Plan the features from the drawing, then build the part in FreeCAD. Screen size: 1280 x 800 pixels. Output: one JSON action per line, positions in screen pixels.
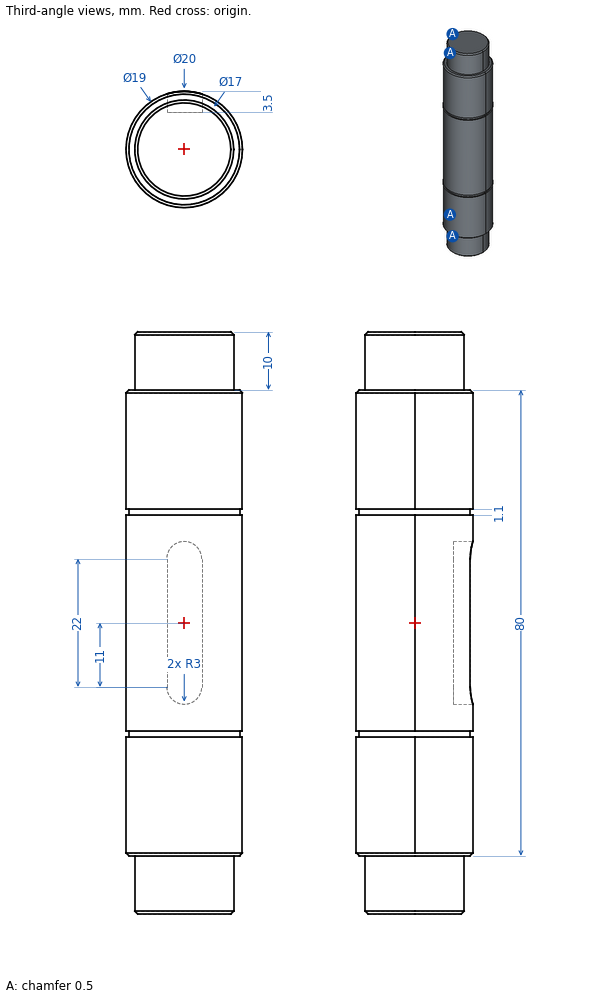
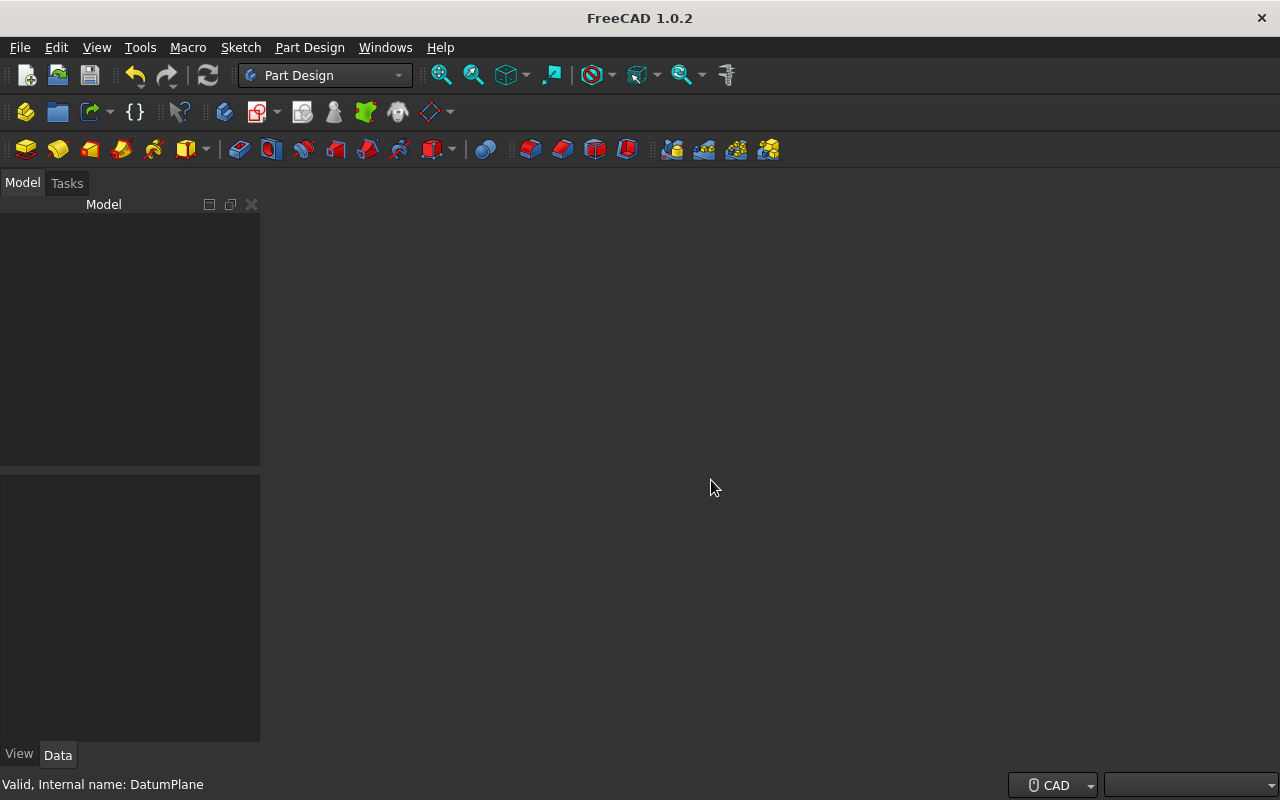
{"action": "left_click", "coordinate": [26, 76]}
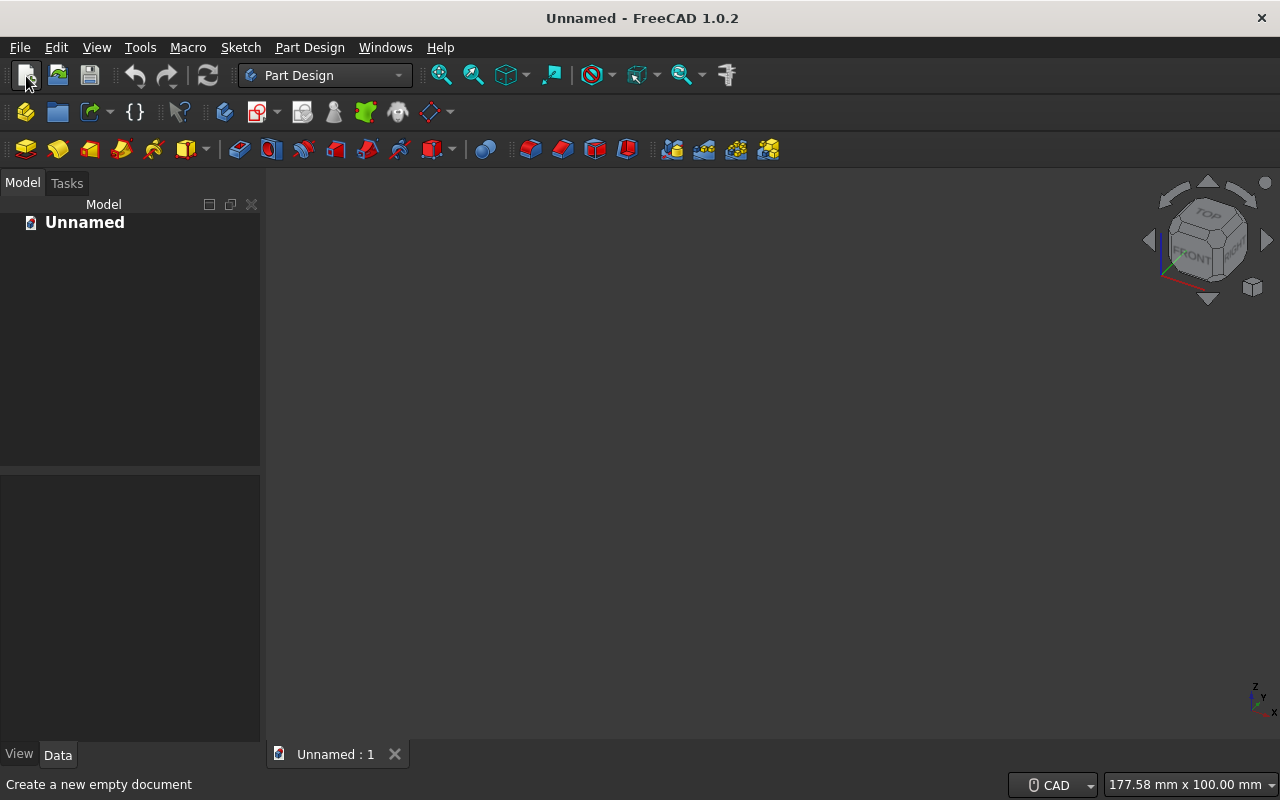
{"action": "left_click", "coordinate": [258, 112]}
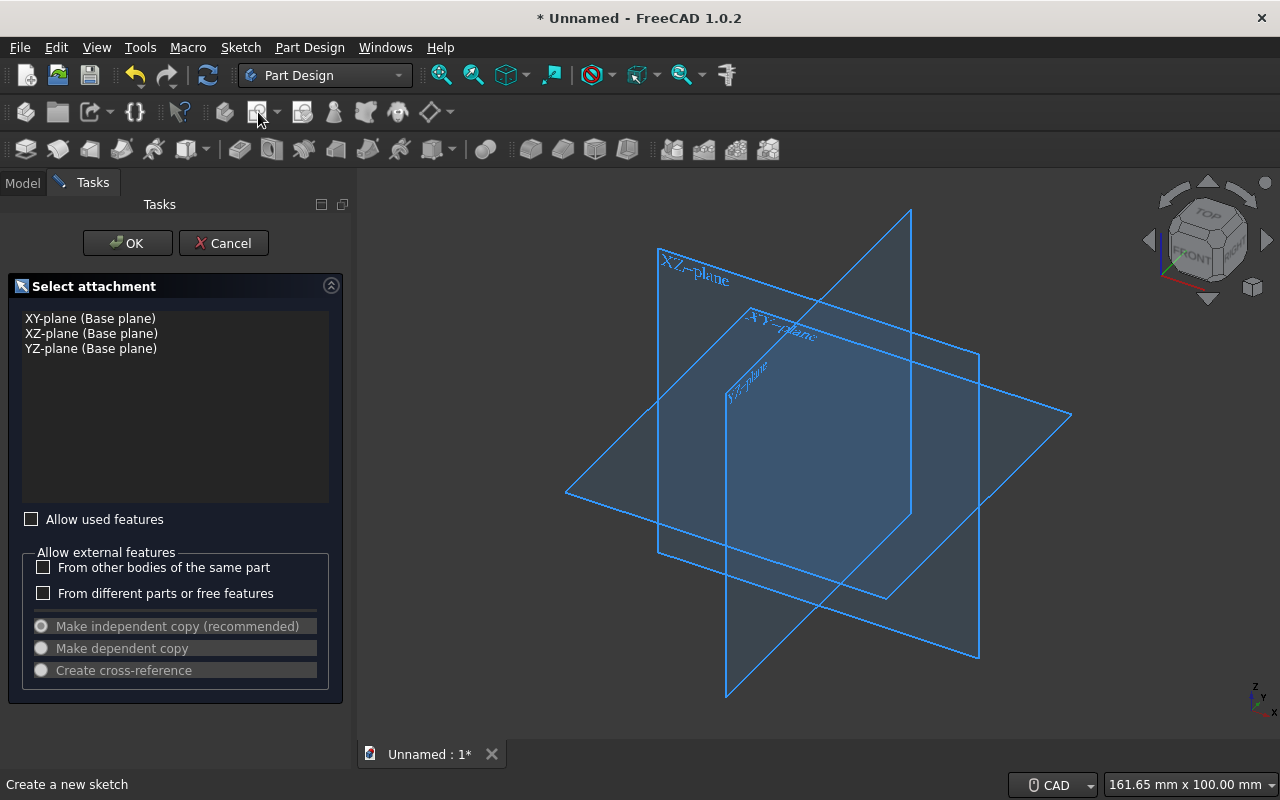
{"action": "left_click", "coordinate": [82, 318]}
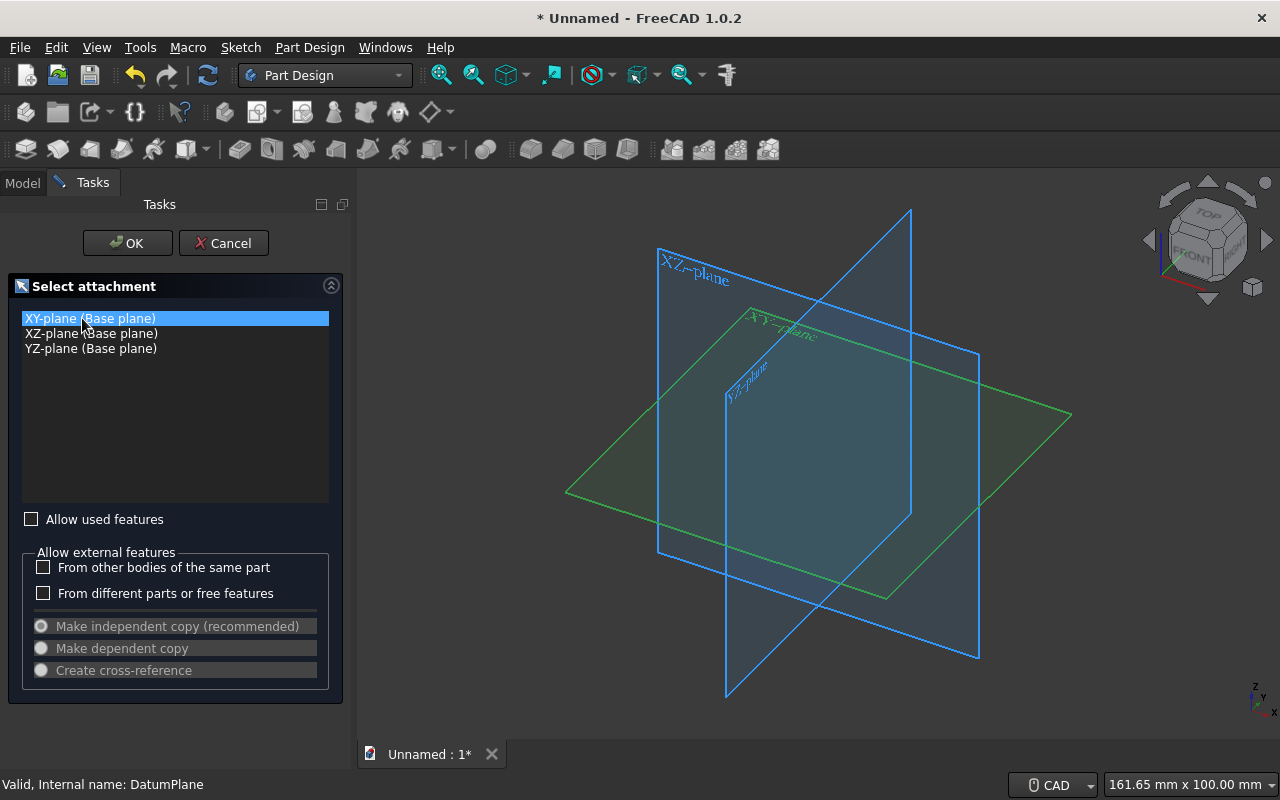
{"action": "left_click", "coordinate": [128, 243]}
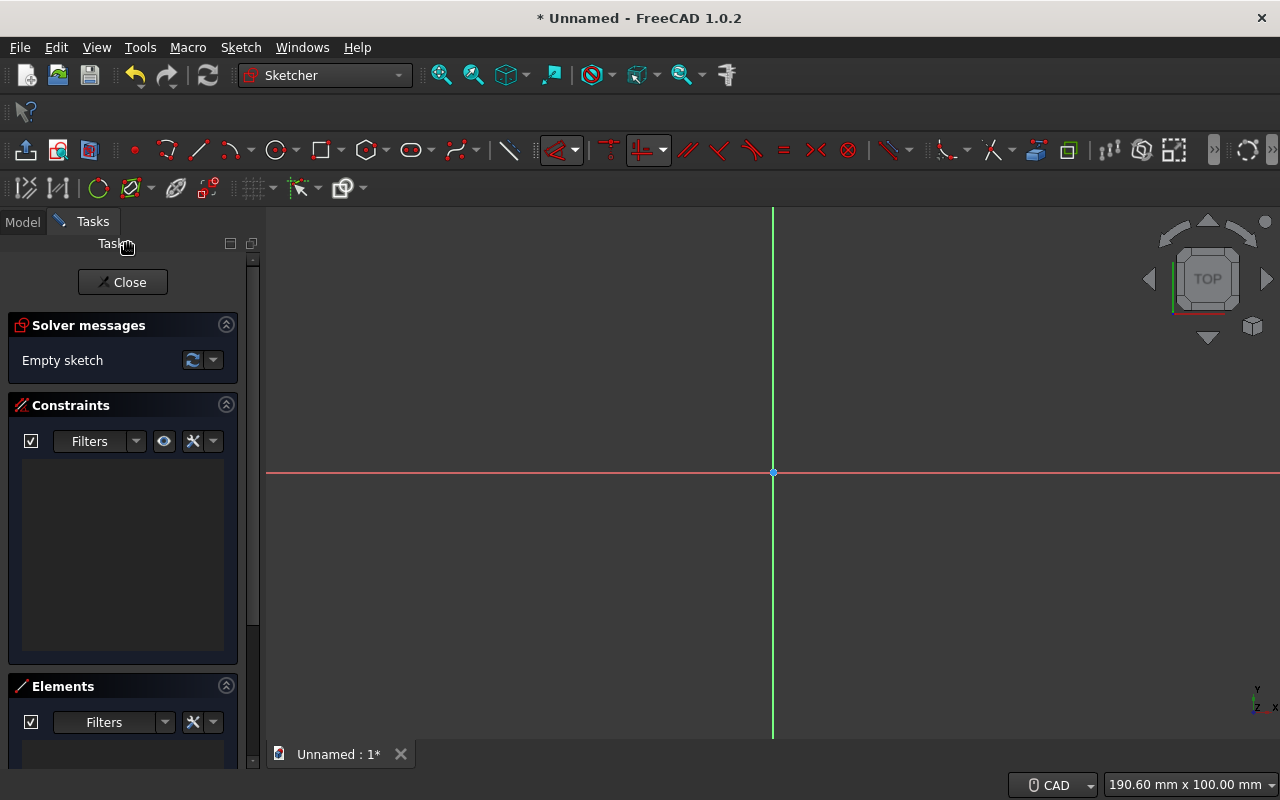
{"action": "scroll", "coordinate": [803, 473], "scroll_direction": "up", "scroll_amount": 6}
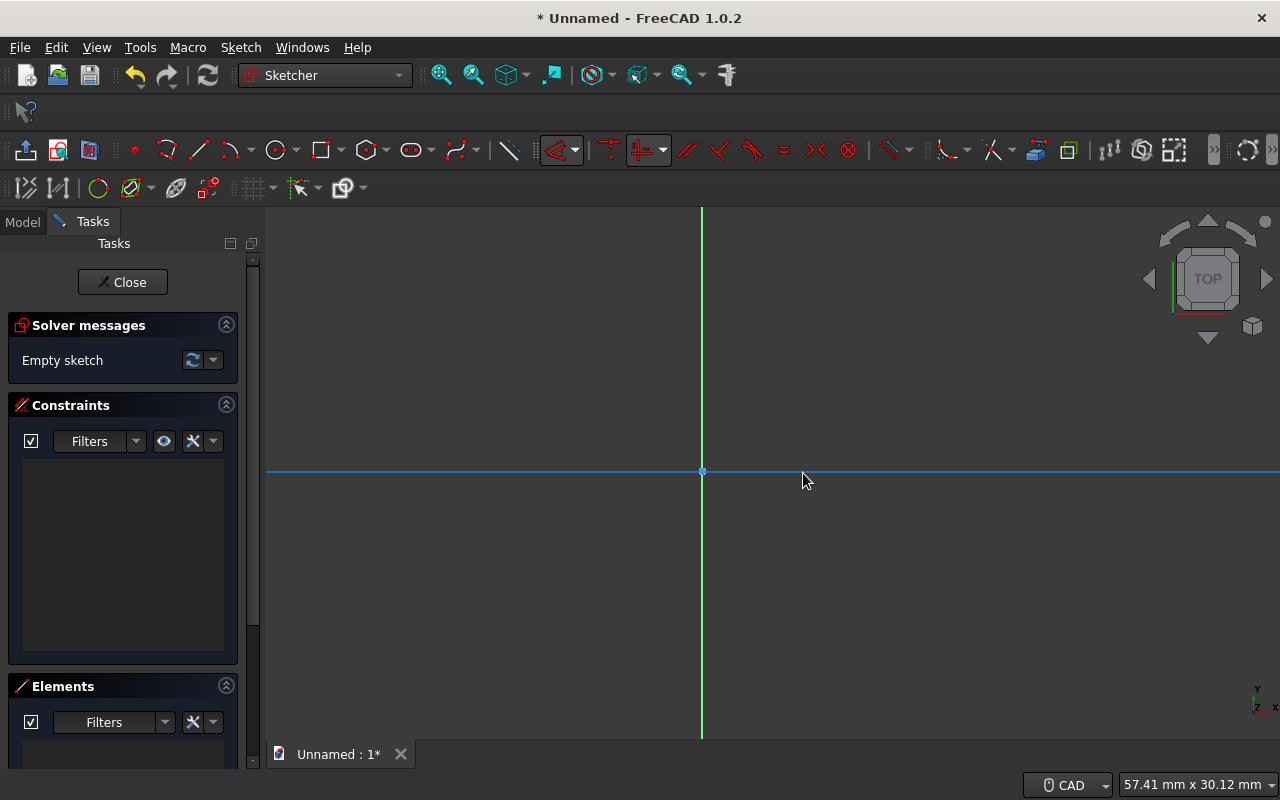
{"action": "key", "text": "g c"}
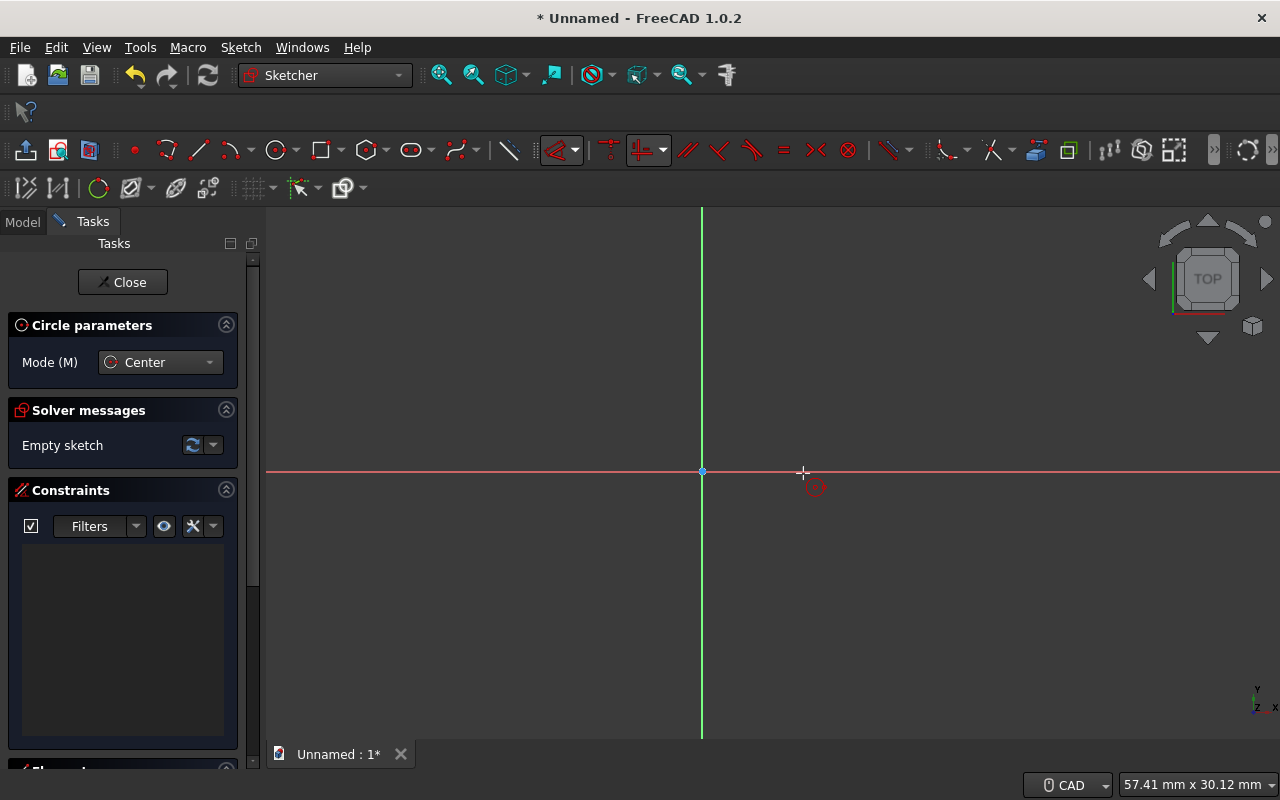
{"action": "left_click", "coordinate": [702, 472]}
{"action": "left_click", "coordinate": [827, 347]}
{"action": "key", "text": "Escape"}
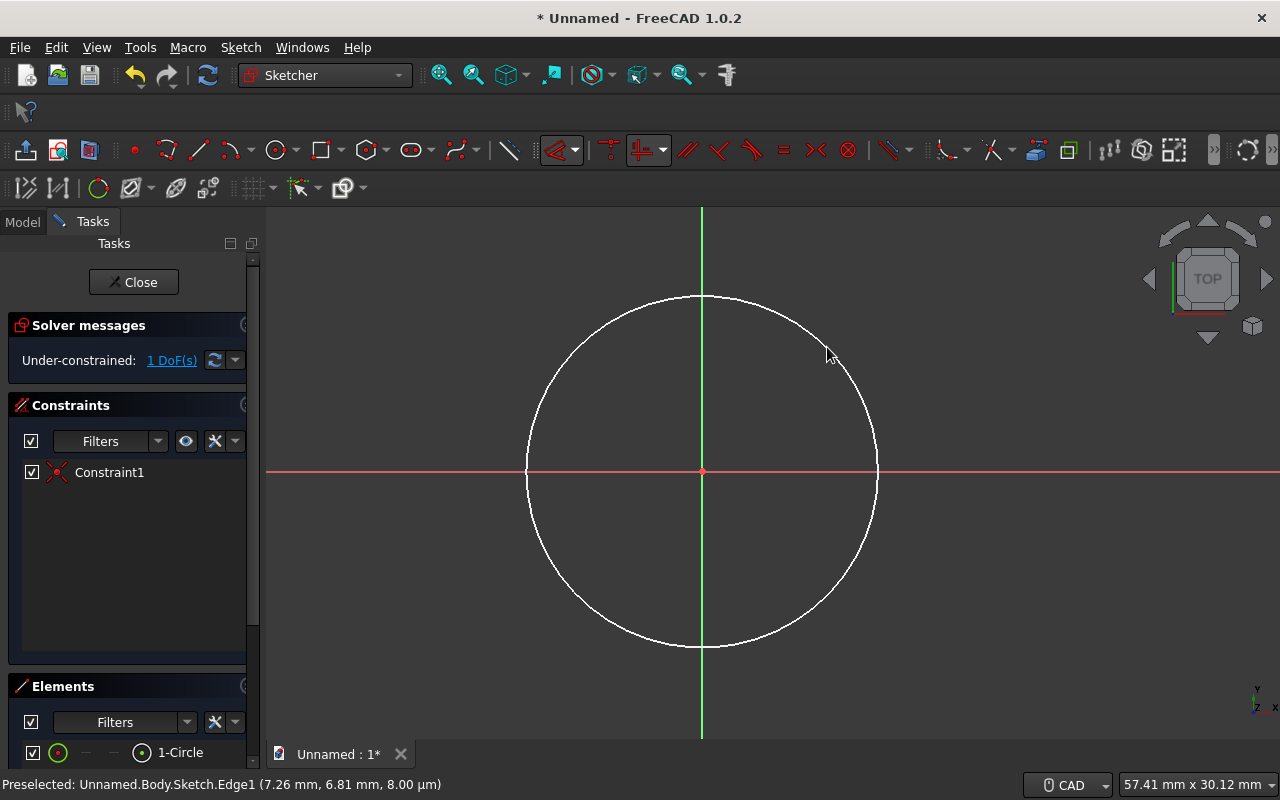
{"action": "key", "text": "d"}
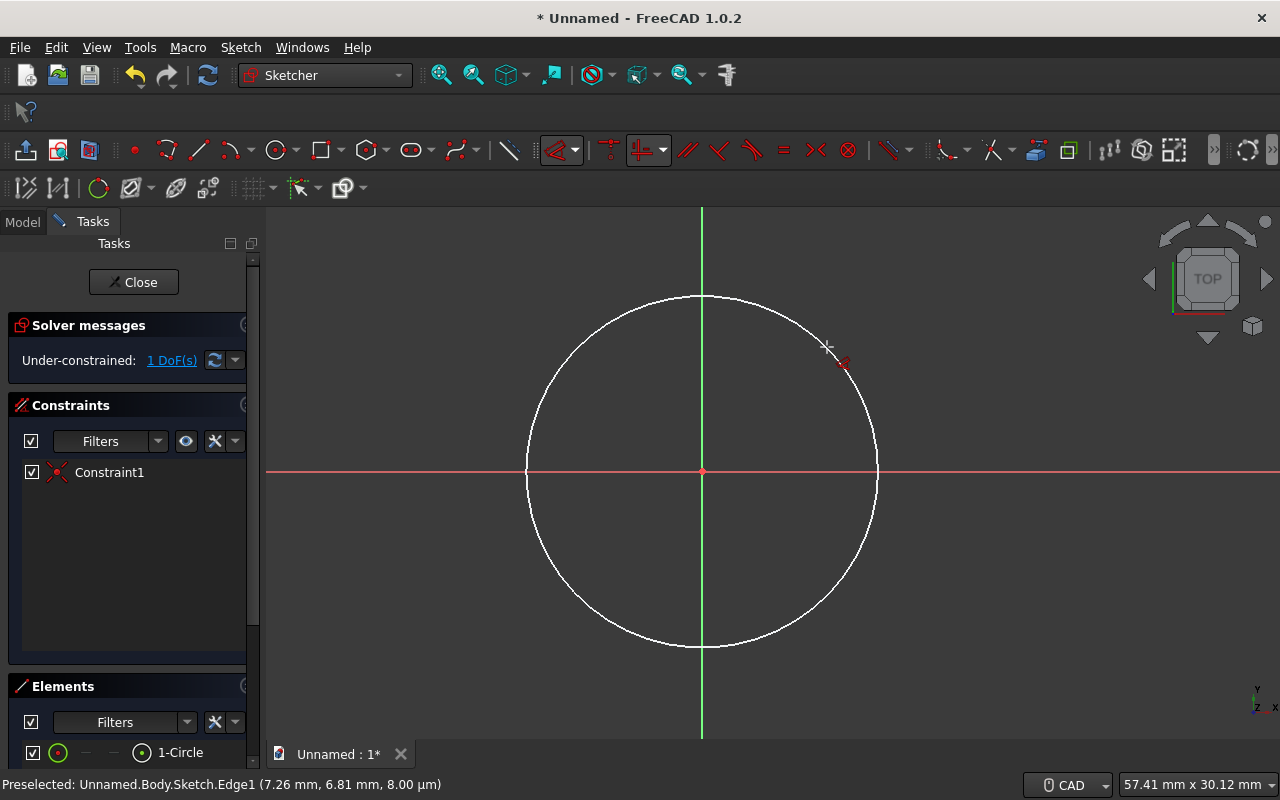
{"action": "left_click", "coordinate": [826, 347]}
{"action": "left_click", "coordinate": [849, 324]}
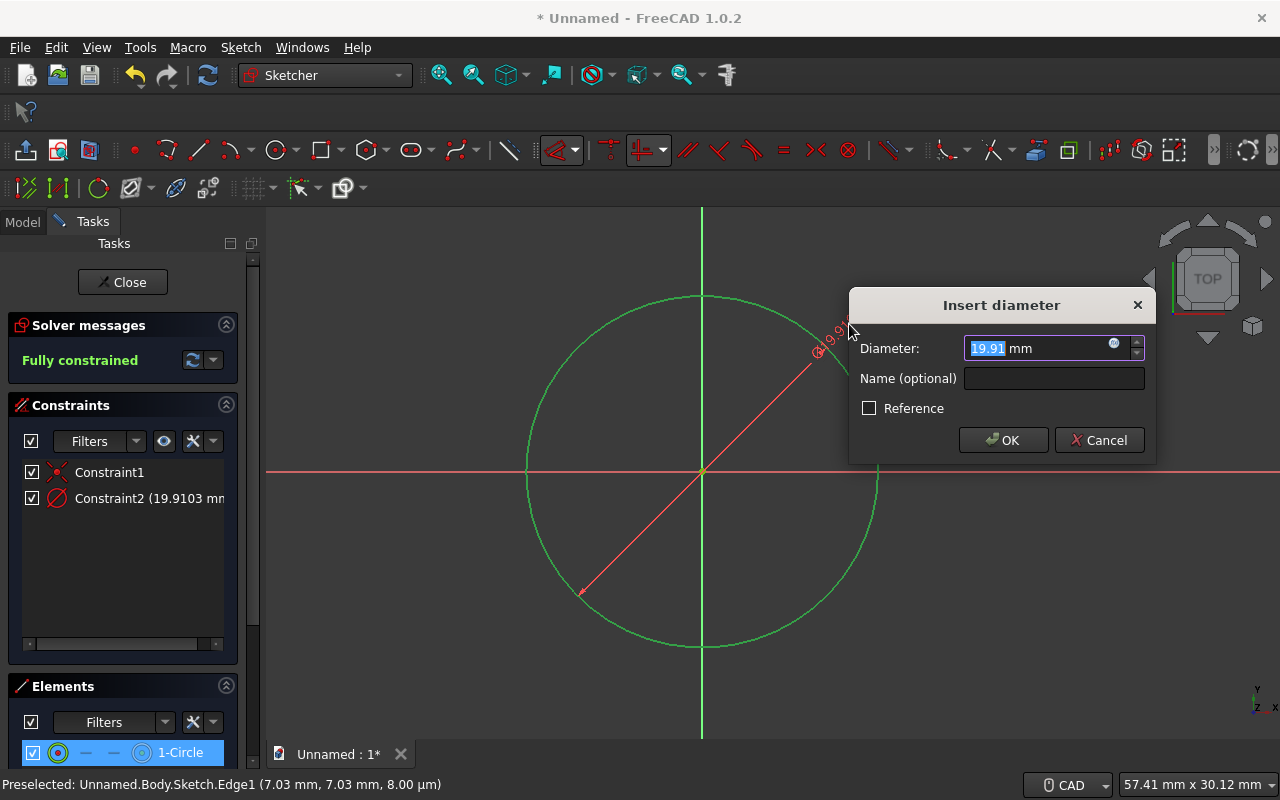
{"action": "type", "text": "20"}
{"action": "key", "text": "Return"}
{"action": "key", "text": "Escape"}